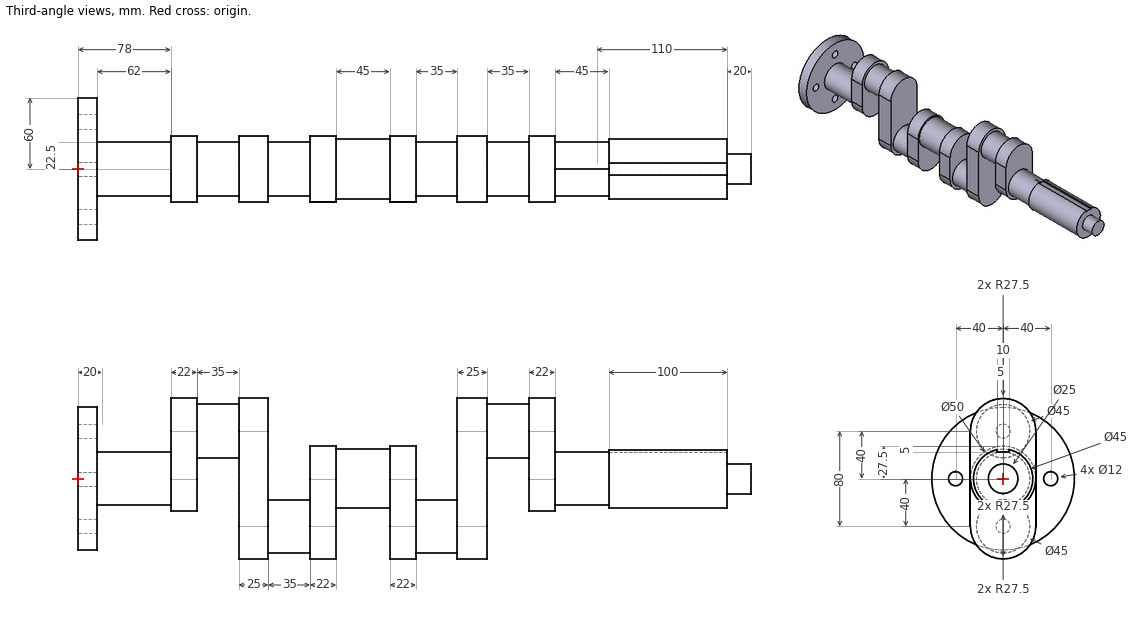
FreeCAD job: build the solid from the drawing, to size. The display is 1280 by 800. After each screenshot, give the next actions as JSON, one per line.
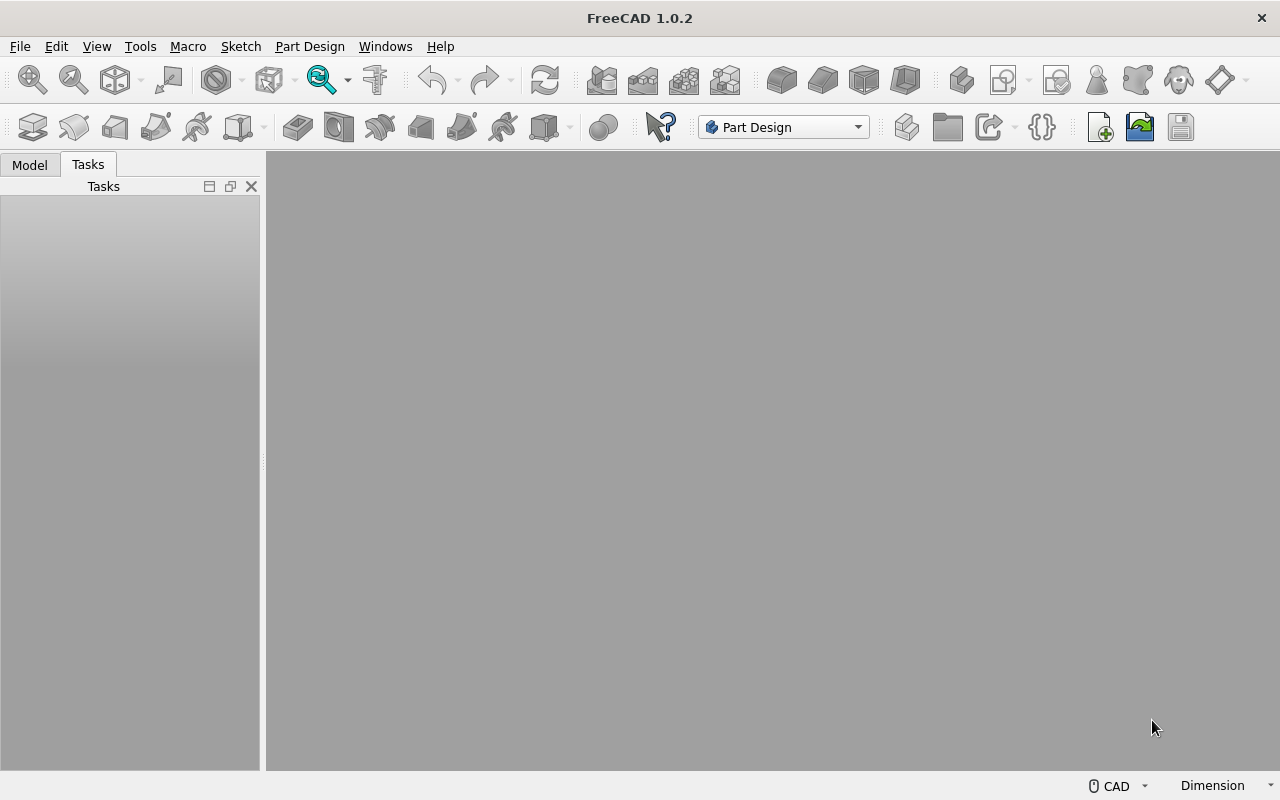
{"action": "key", "text": "ctrl+n"}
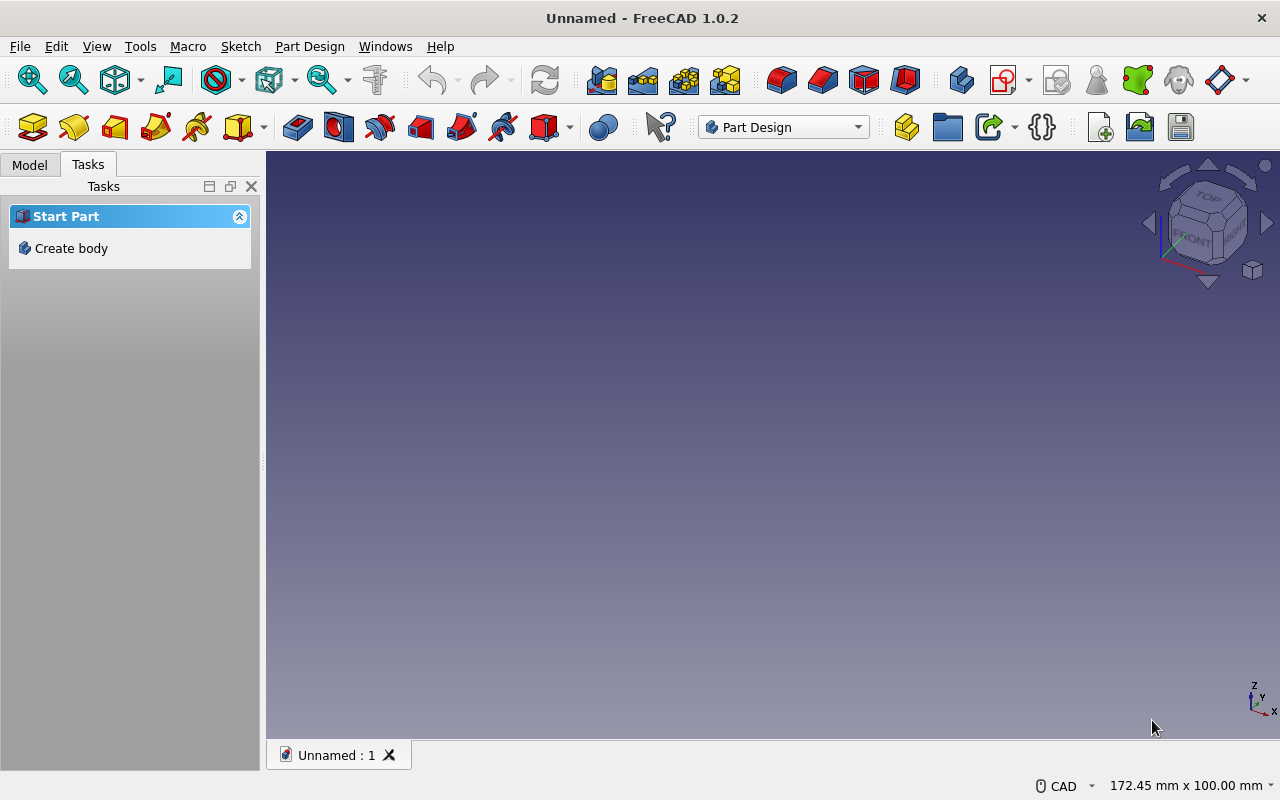
{"action": "left_click", "coordinate": [1002, 80]}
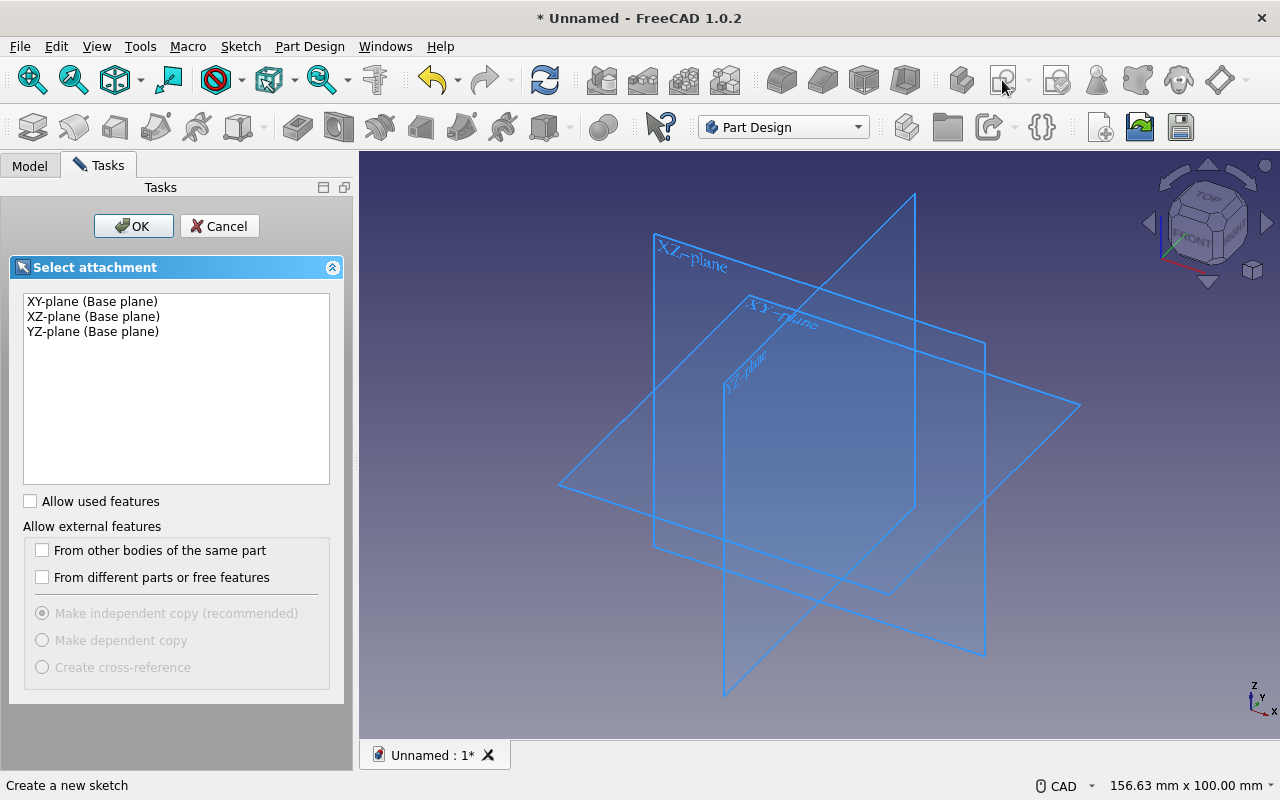
{"action": "left_click", "coordinate": [84, 302]}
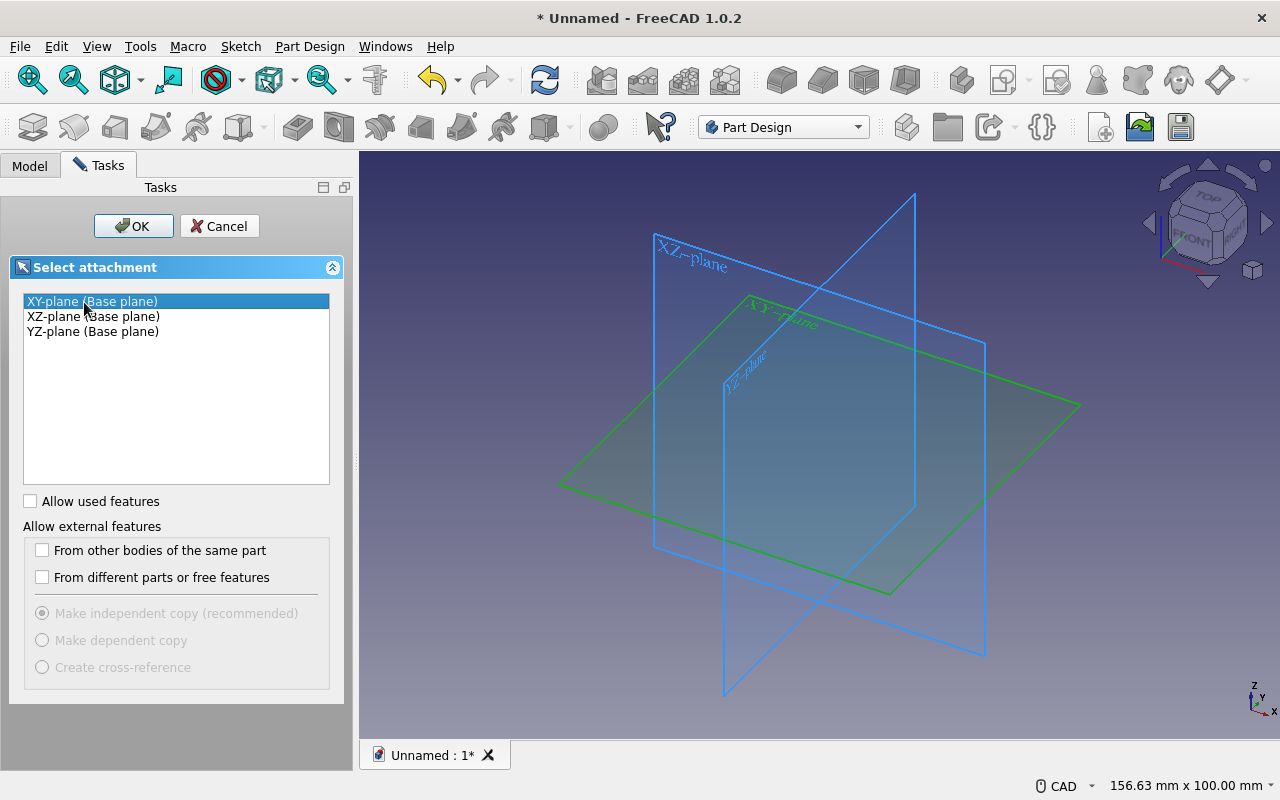
{"action": "left_click", "coordinate": [134, 226]}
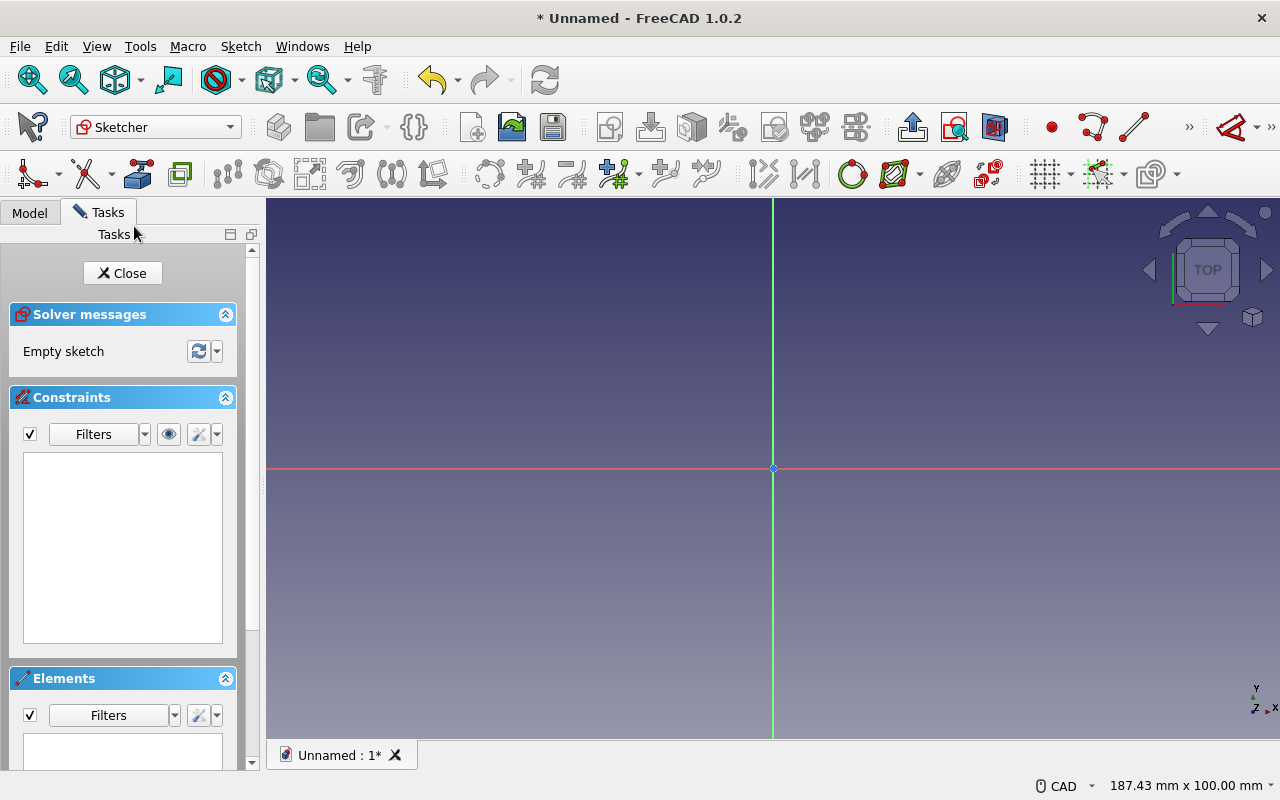
{"action": "scroll", "coordinate": [294, 711], "scroll_direction": "down", "scroll_amount": 2}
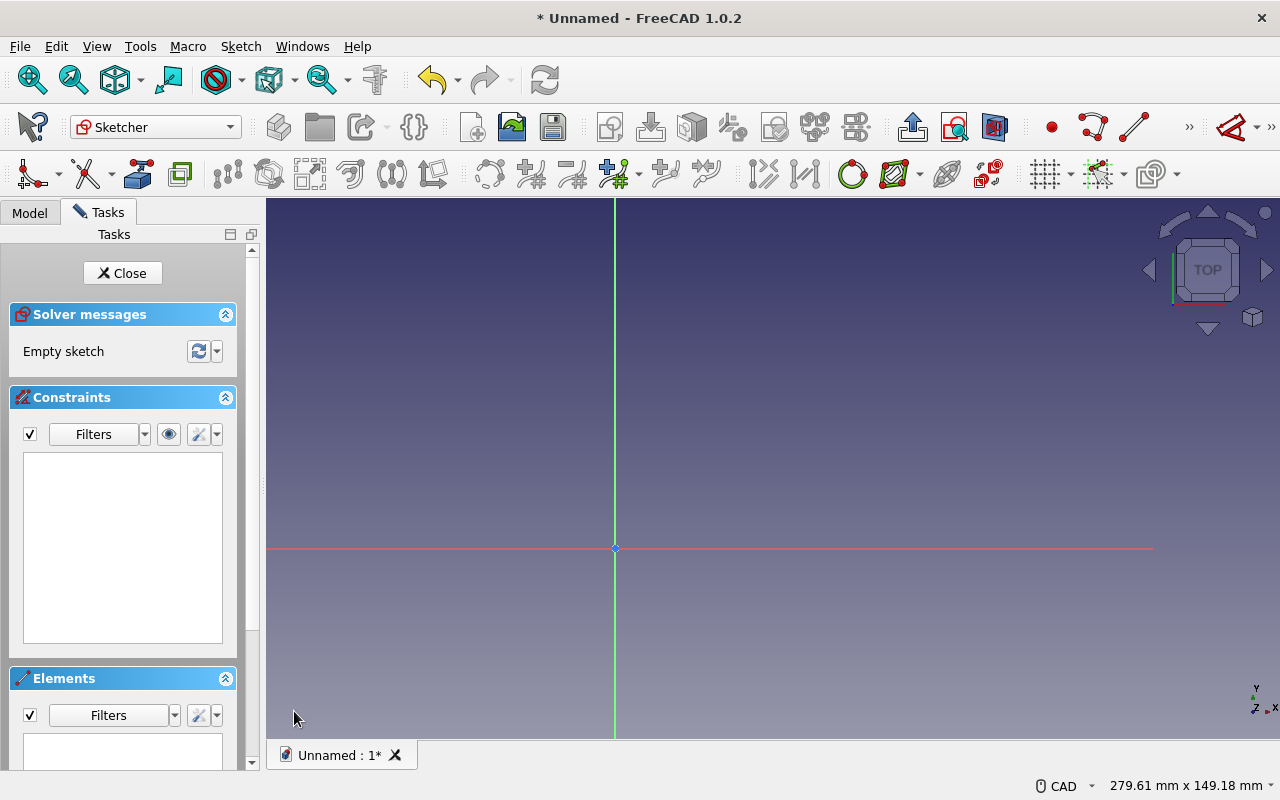
{"action": "scroll", "coordinate": [862, 382], "scroll_direction": "up", "scroll_amount": 2}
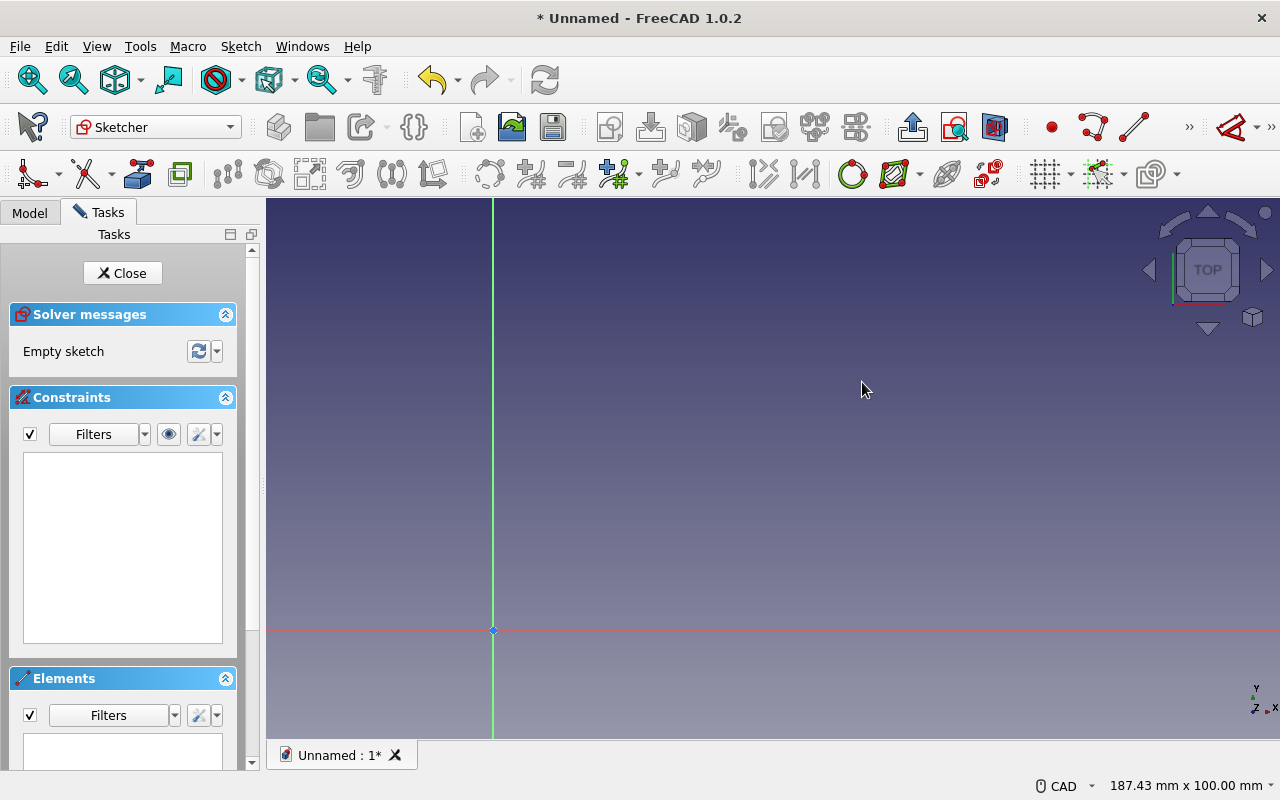
{"action": "left_click", "coordinate": [1093, 128]}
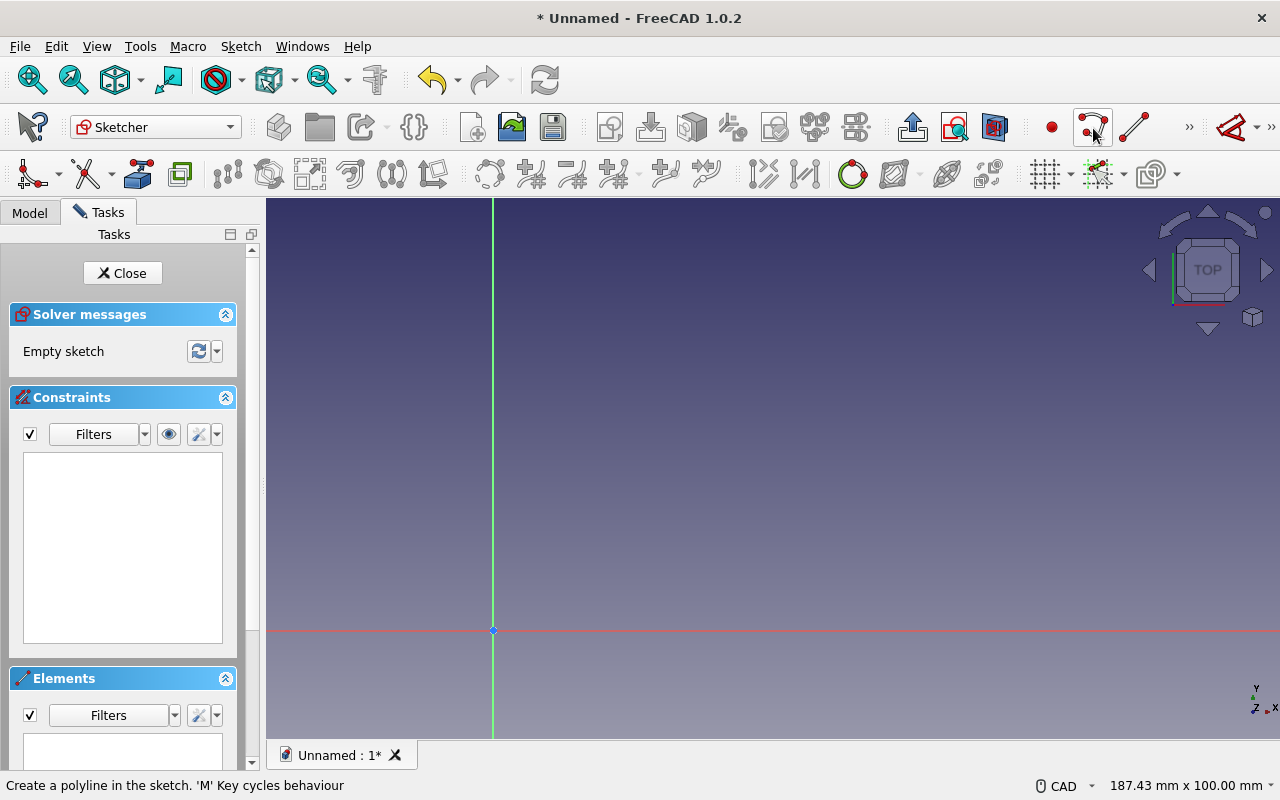
{"action": "left_click", "coordinate": [493, 631]}
{"action": "left_click", "coordinate": [915, 622]}
{"action": "left_click", "coordinate": [915, 509]}
{"action": "left_click", "coordinate": [580, 509]}
{"action": "left_click", "coordinate": [580, 306]}
{"action": "left_click", "coordinate": [502, 306]}
{"action": "left_click", "coordinate": [493, 631]}
{"action": "key", "text": "Escape"}
{"action": "key", "text": "Escape"}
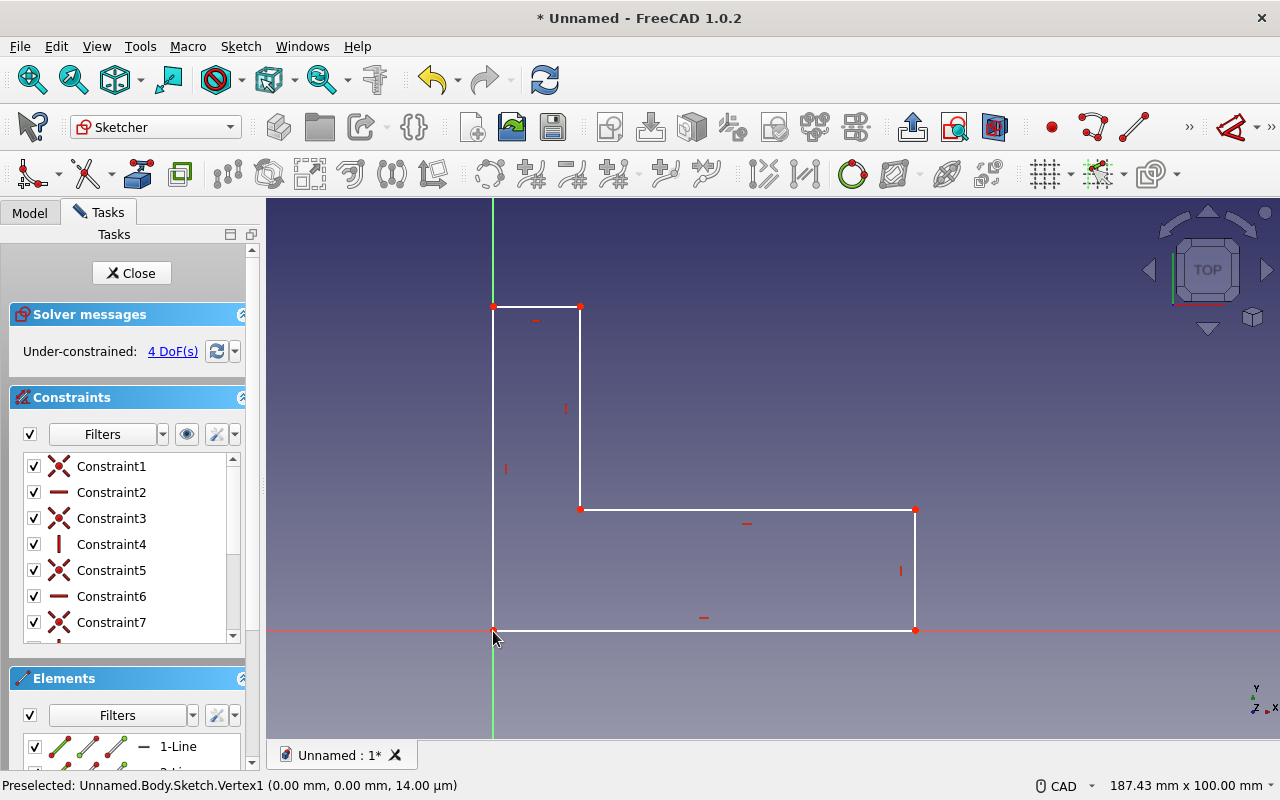
{"action": "left_click", "coordinate": [1230, 128]}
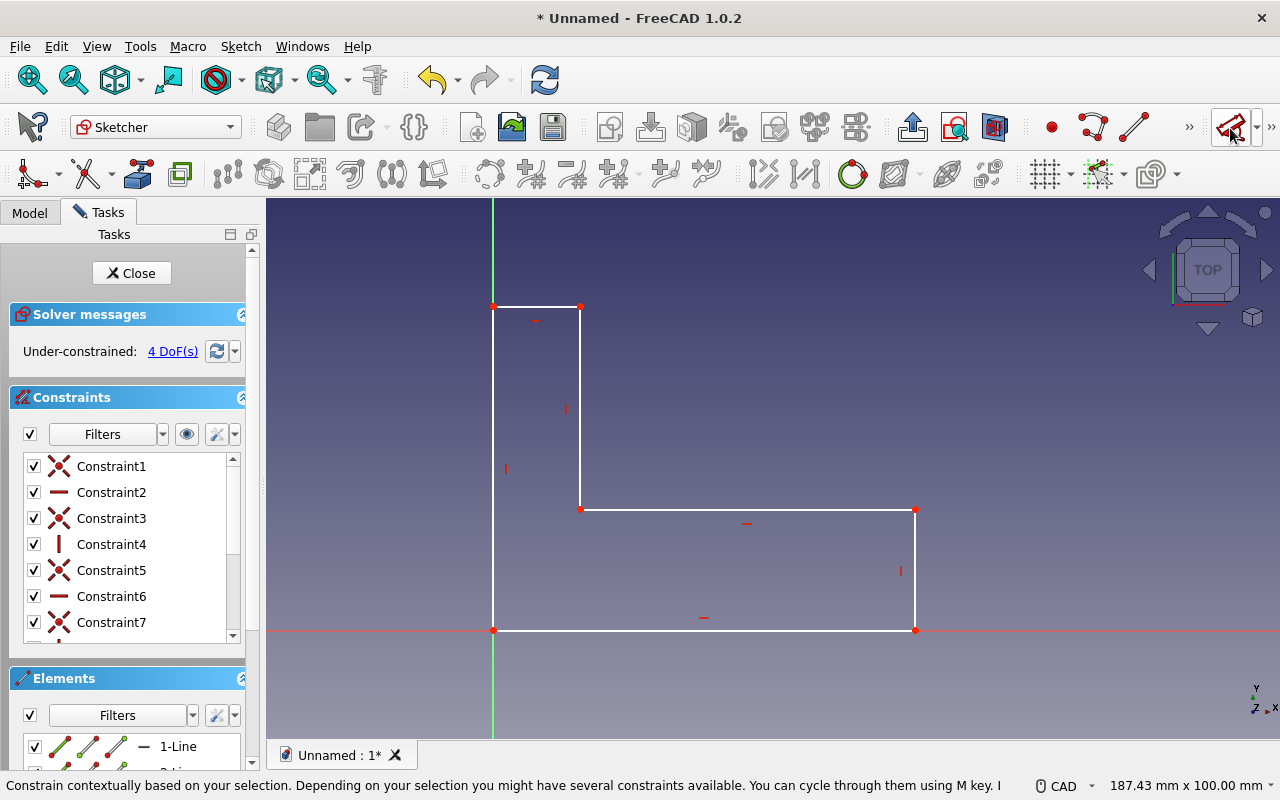
{"action": "left_click", "coordinate": [620, 631]}
{"action": "left_click", "coordinate": [704, 665]}